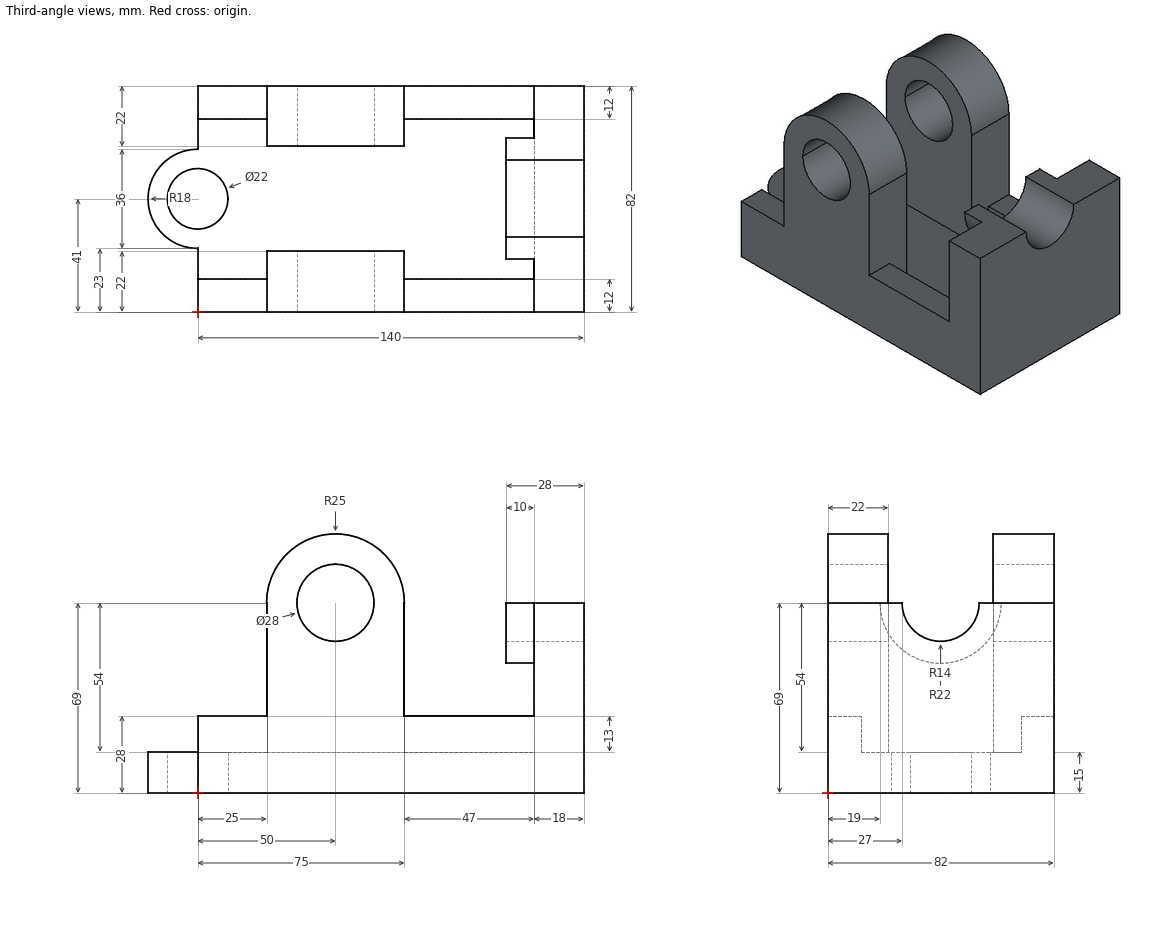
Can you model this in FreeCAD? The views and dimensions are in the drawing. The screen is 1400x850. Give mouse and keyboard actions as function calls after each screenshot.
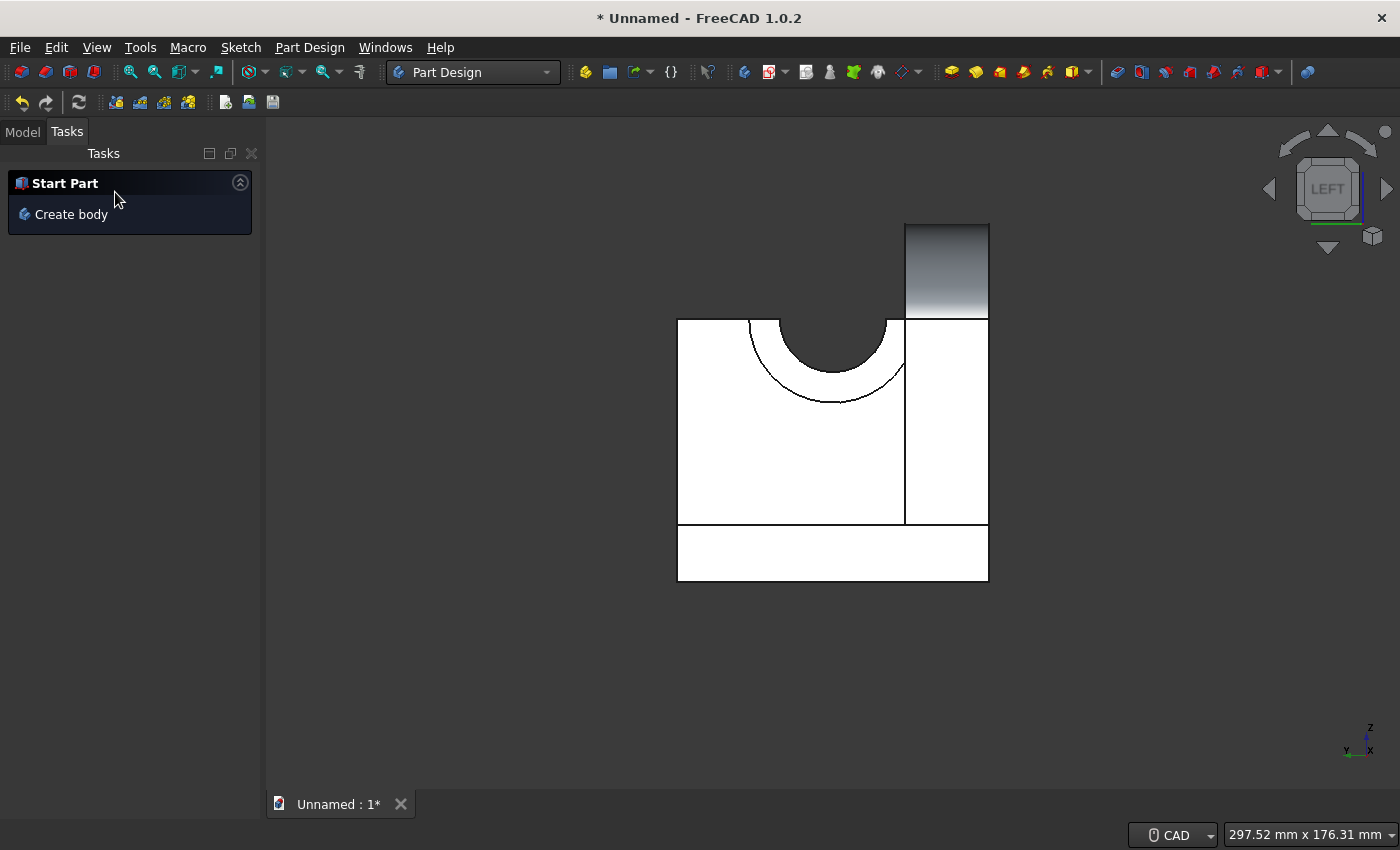
key(0)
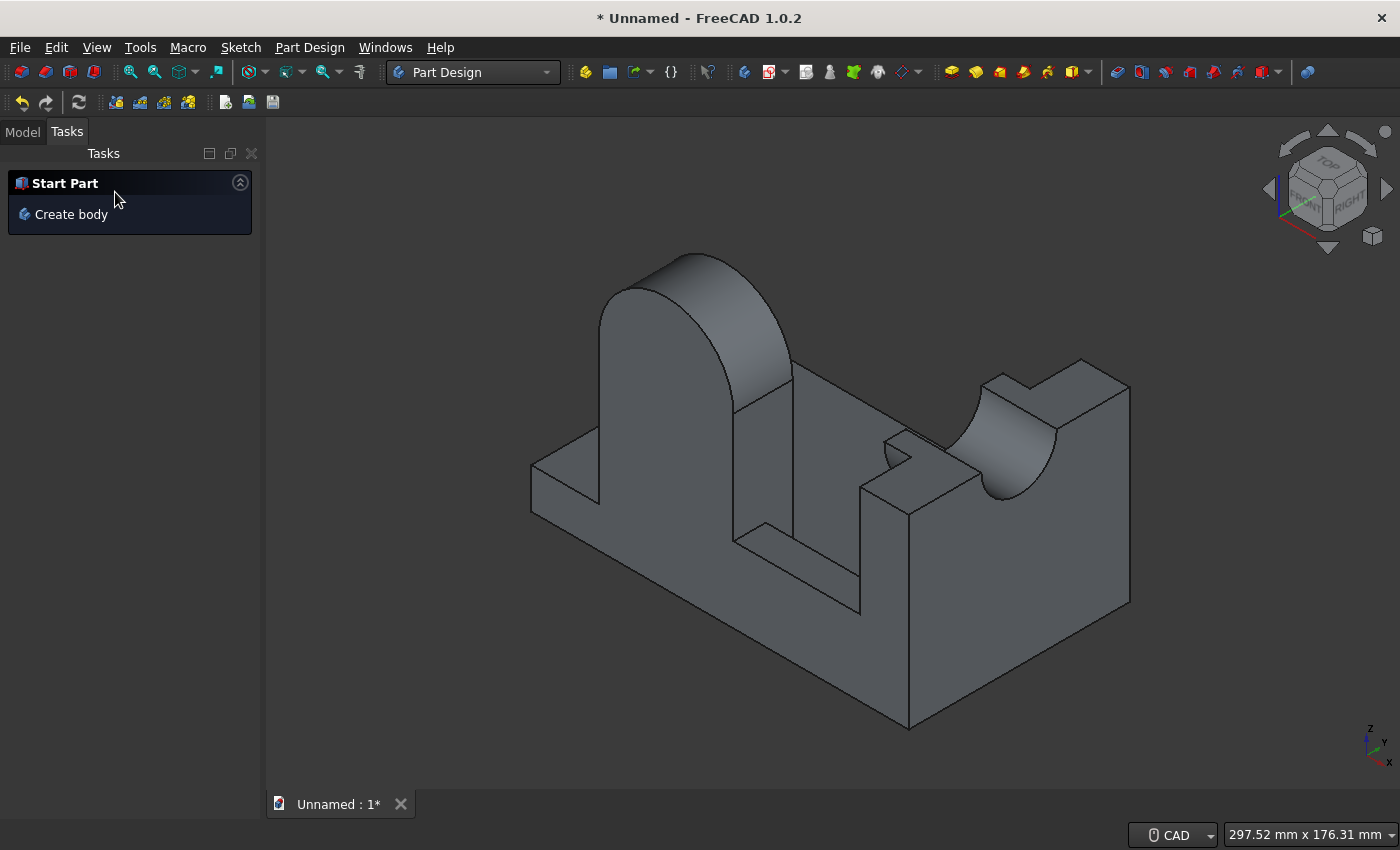
click(132, 72)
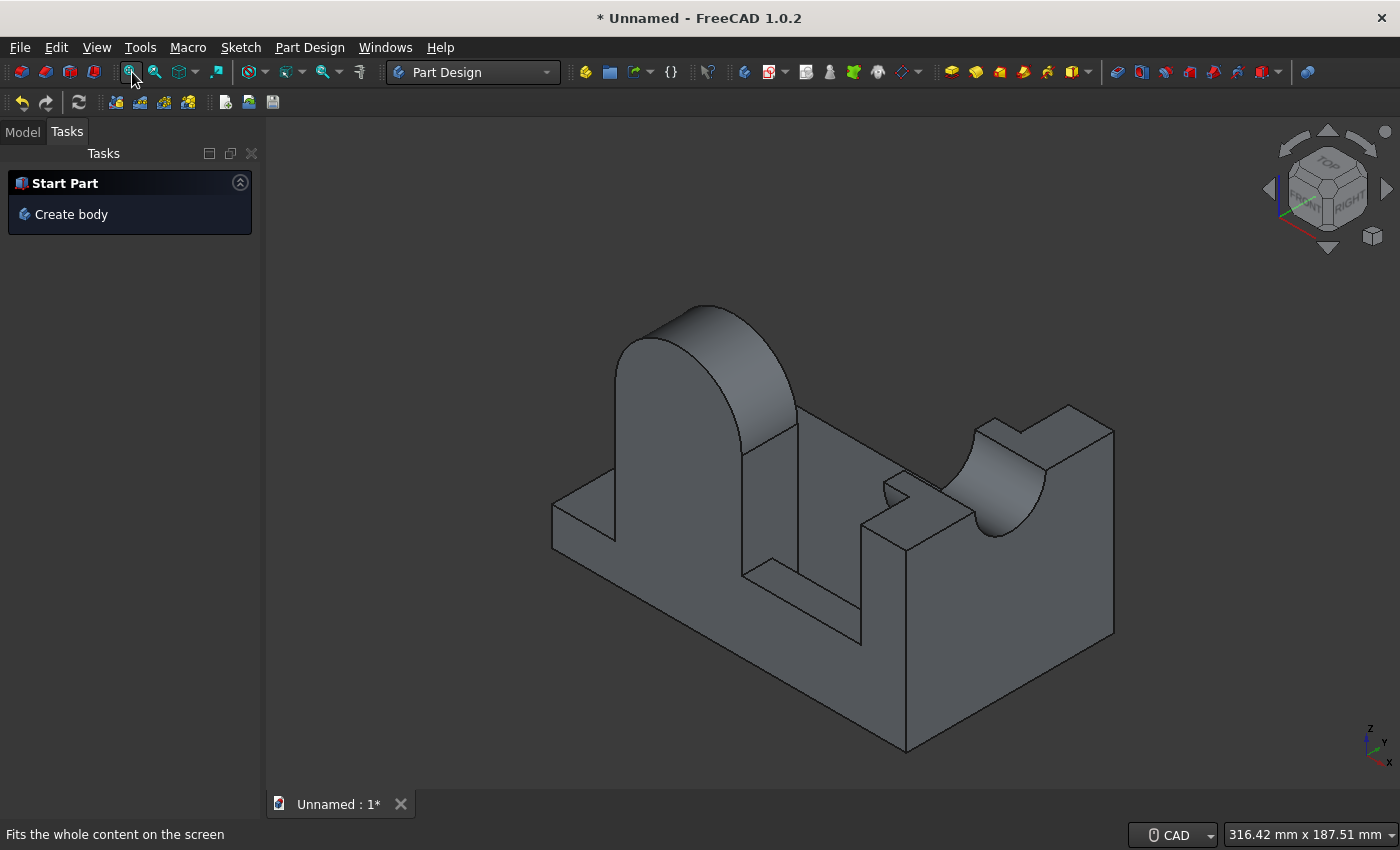
click(678, 443)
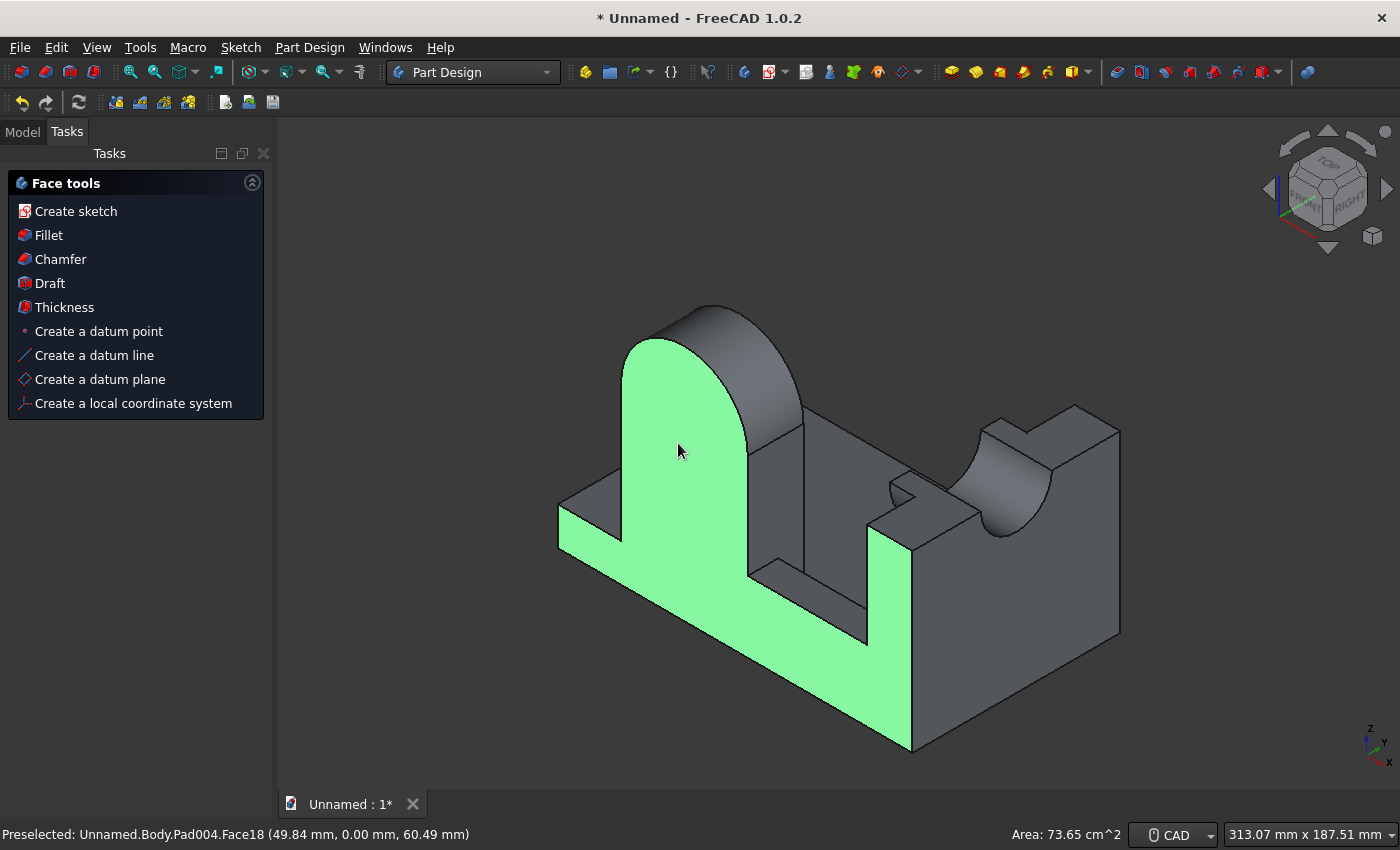
click(770, 72)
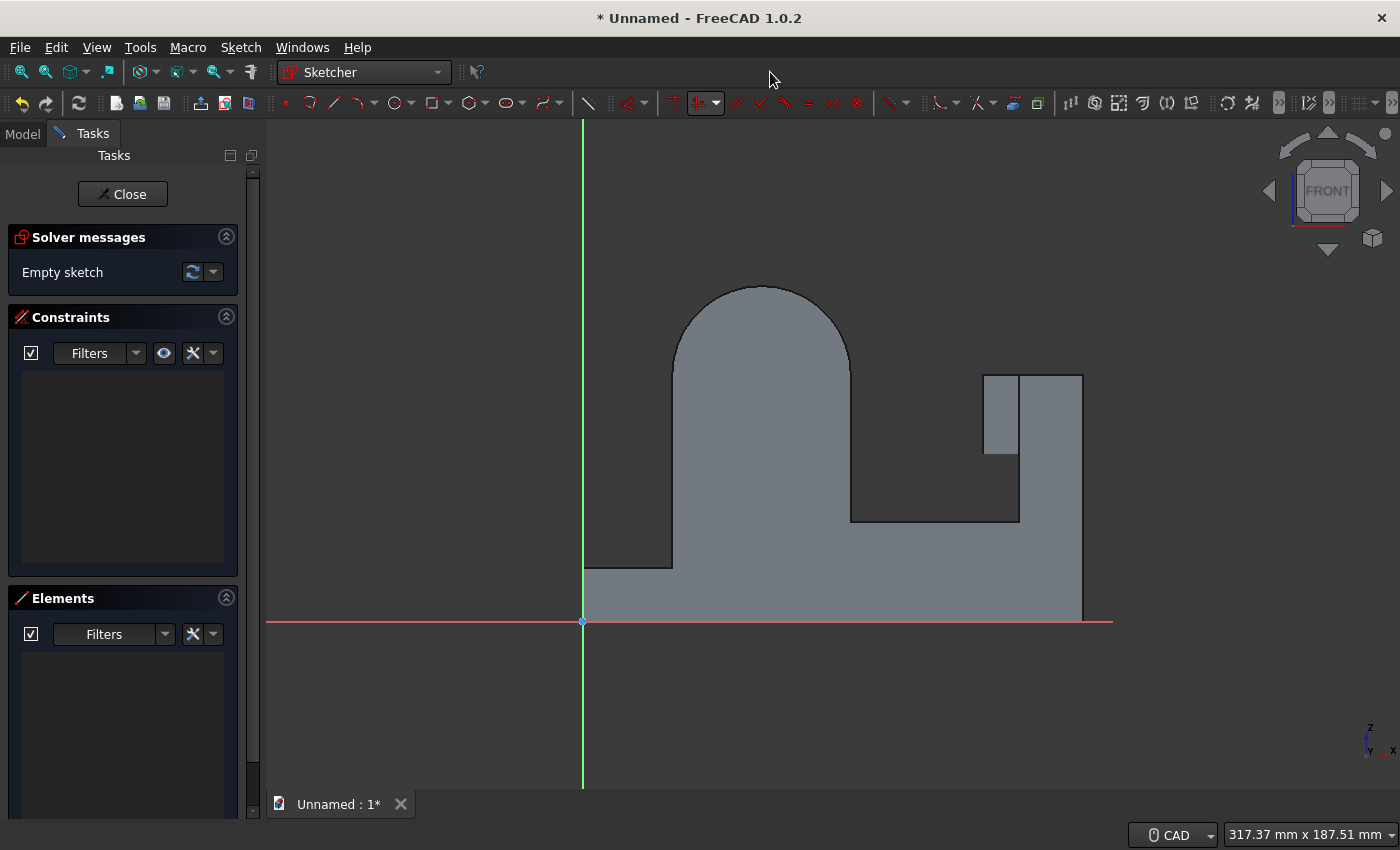
scroll(583, 611, up, 7)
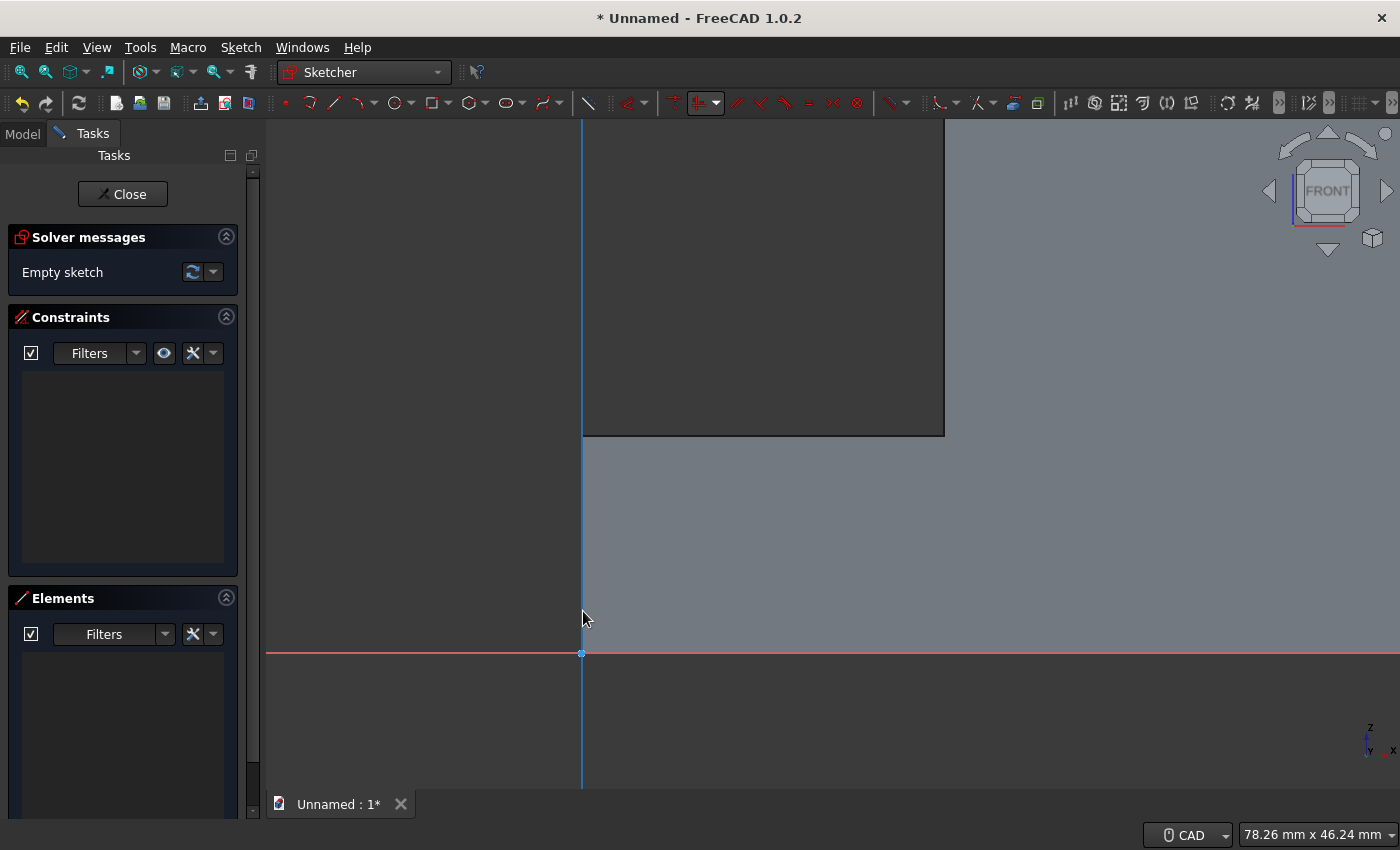
click(432, 104)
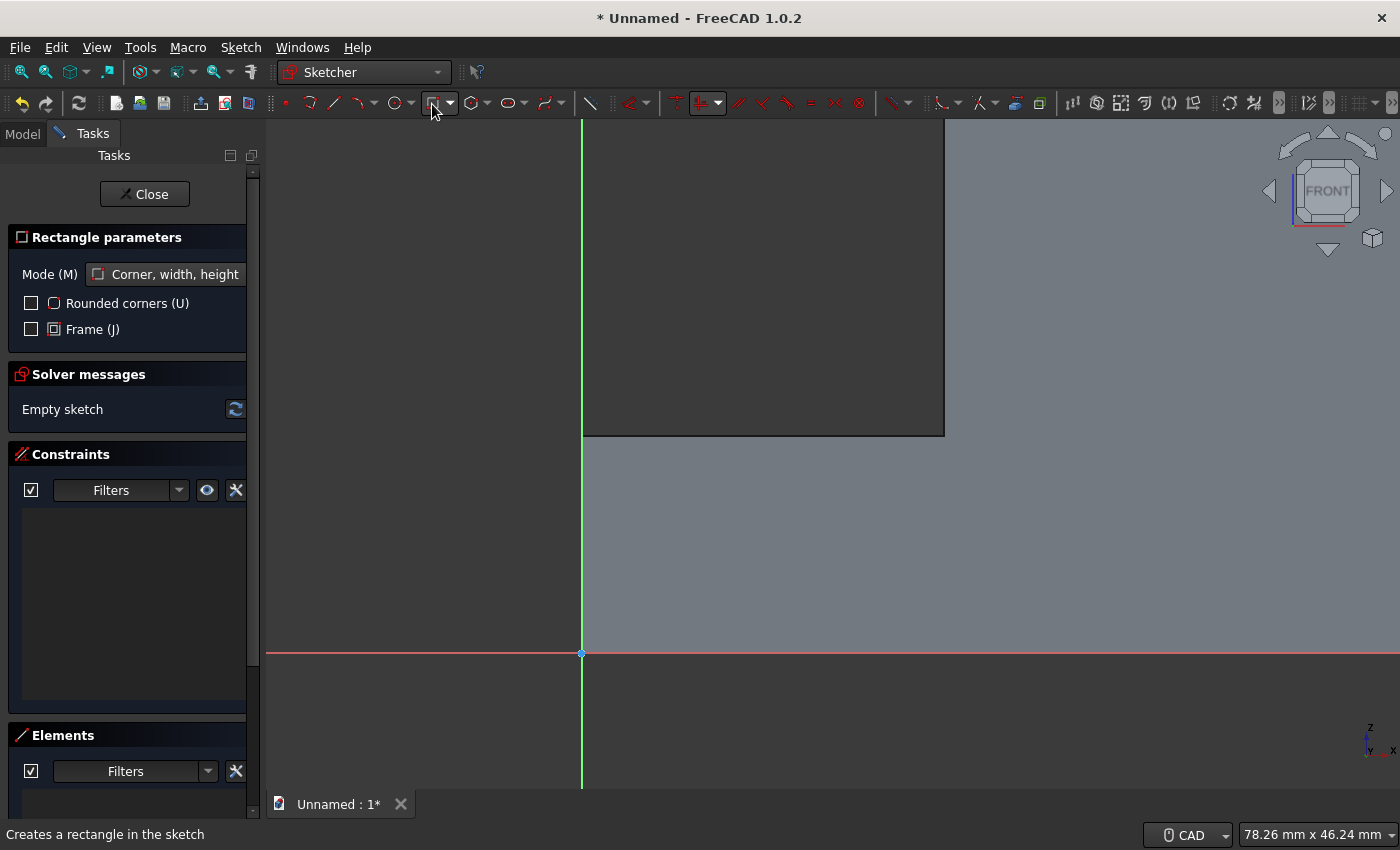
click(582, 247)
click(944, 436)
key(Escape)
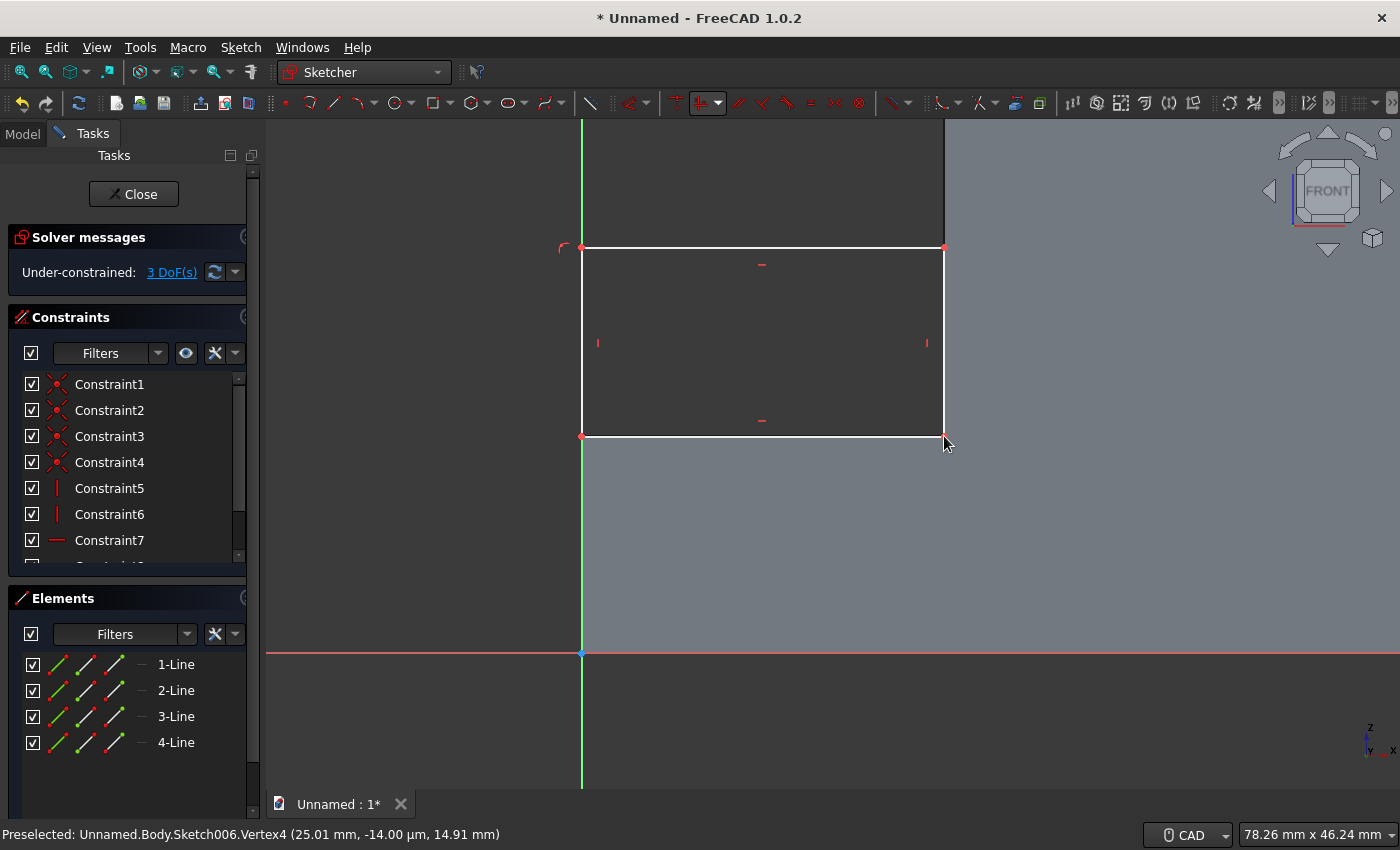
click(630, 104)